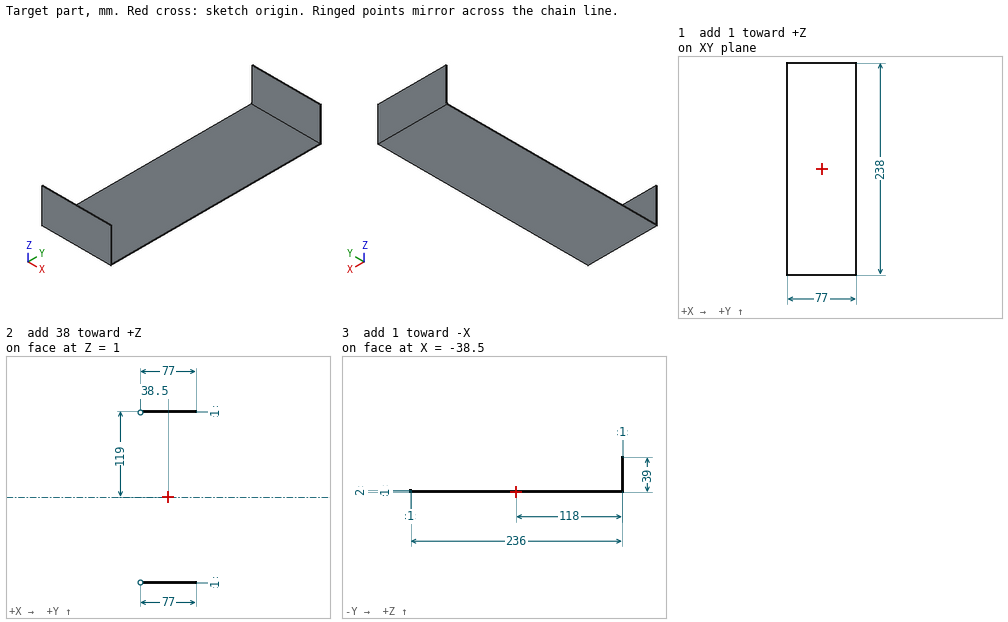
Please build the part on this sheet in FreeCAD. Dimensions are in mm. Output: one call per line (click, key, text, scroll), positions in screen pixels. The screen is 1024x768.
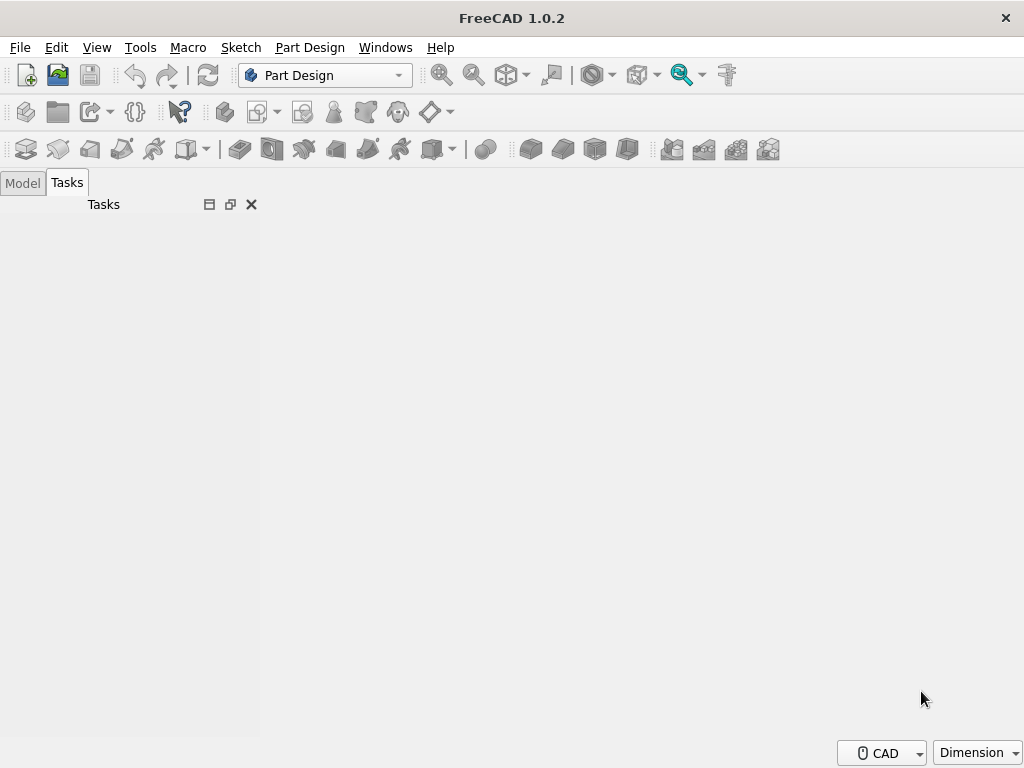
click(26, 76)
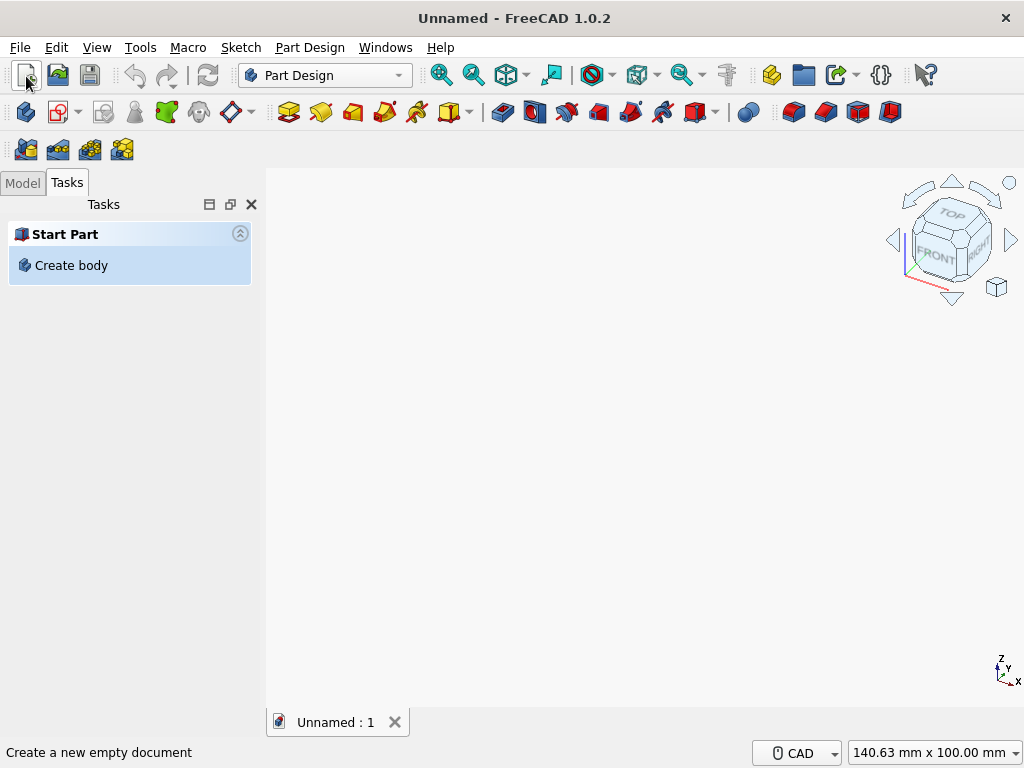
click(58, 112)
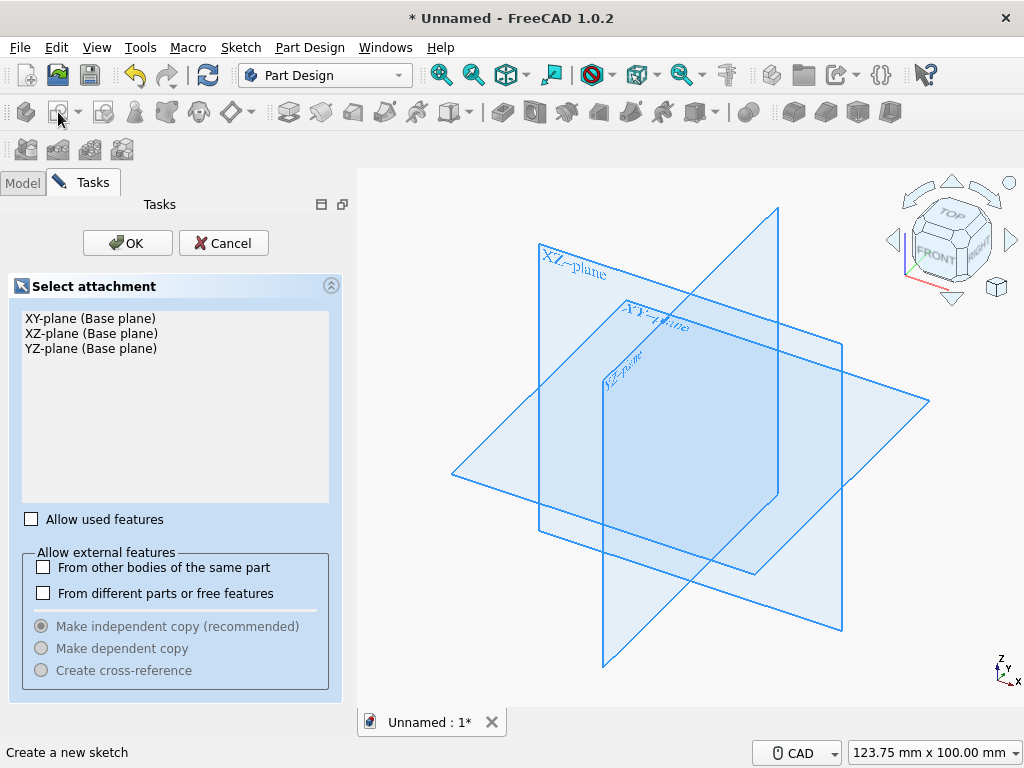
click(82, 318)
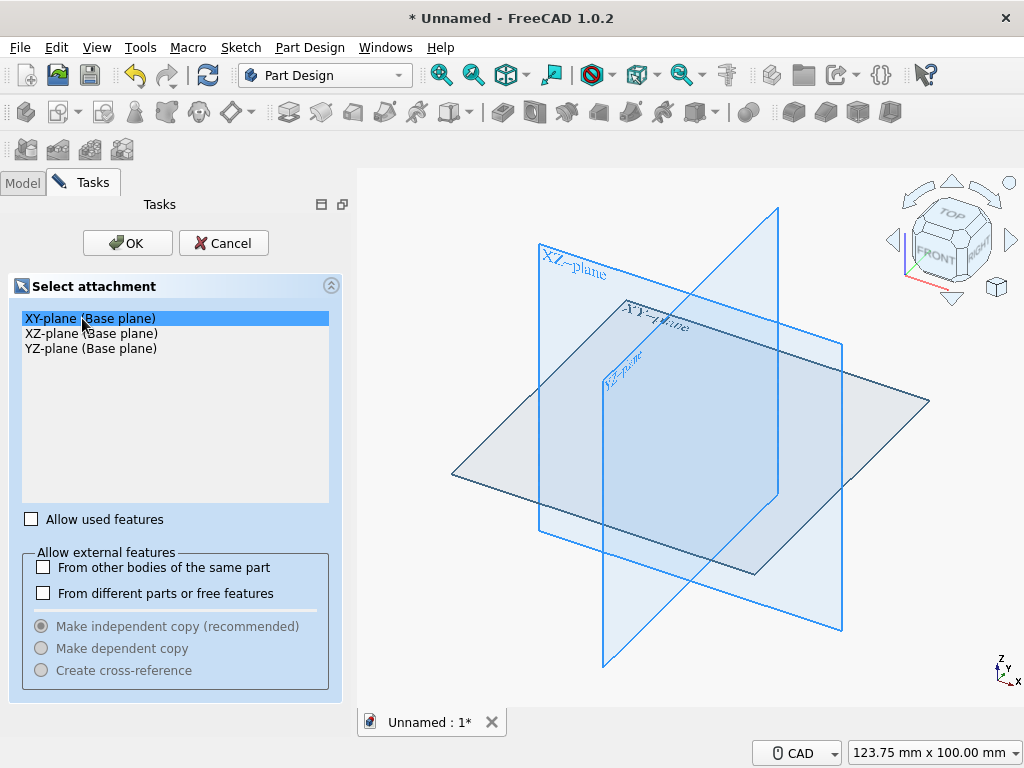
click(128, 243)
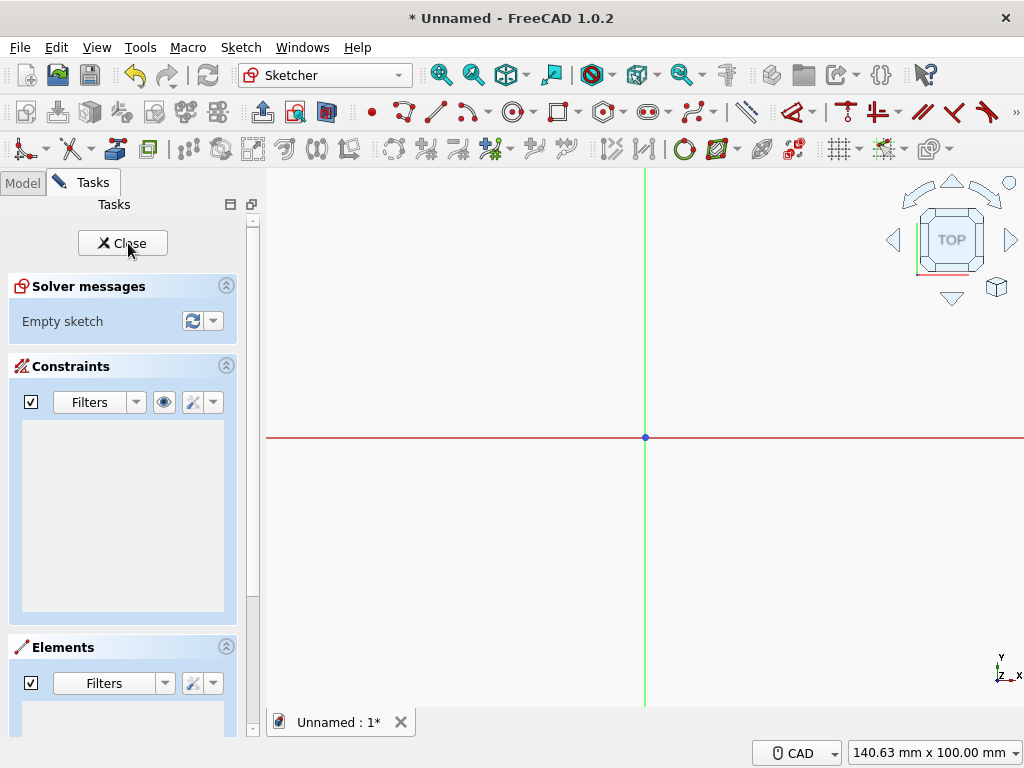
scroll(554, 438, down, 7)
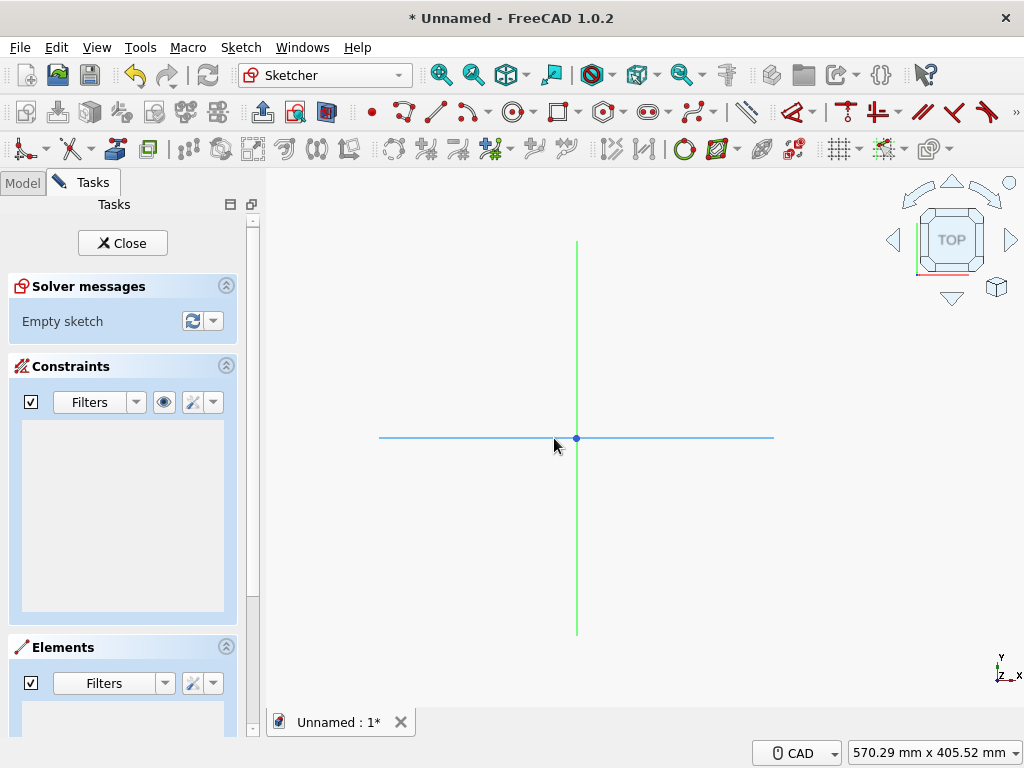
key(g)
key(v)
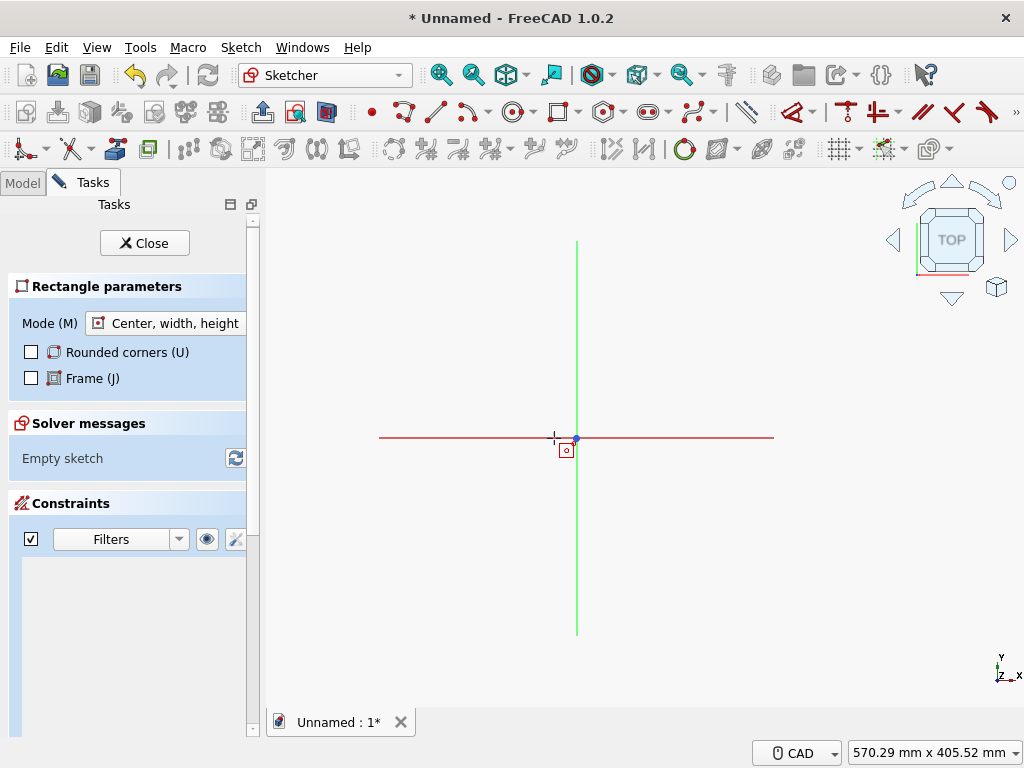
click(577, 438)
move(628, 280)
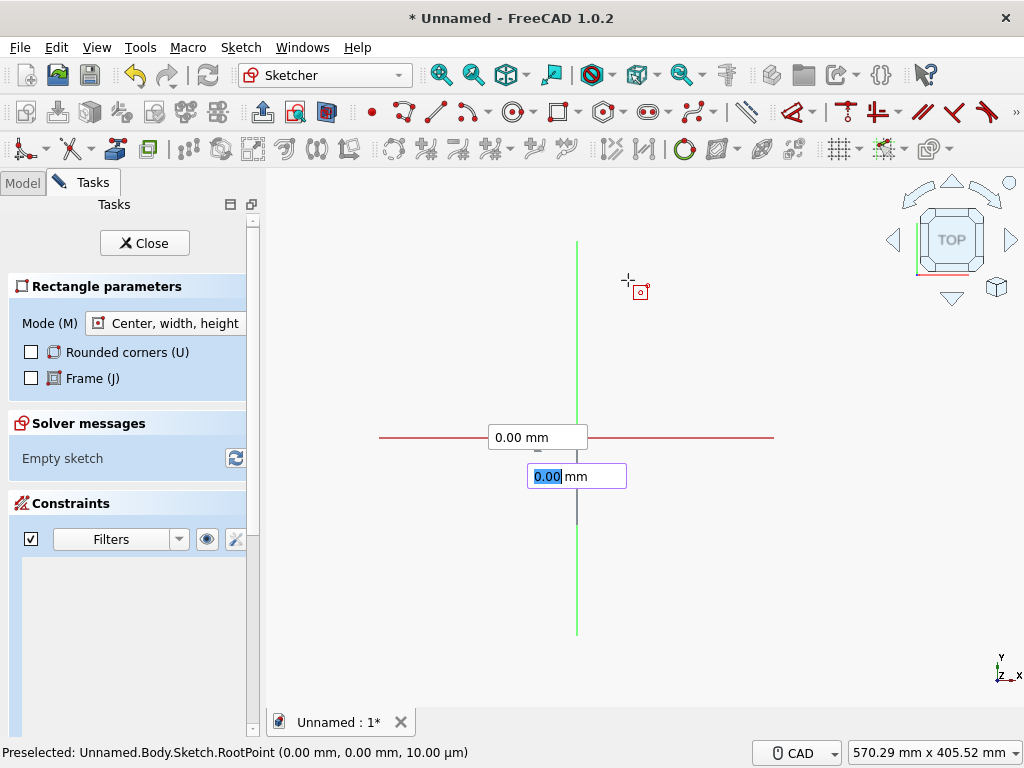
text(77)
key(Tab)
text(238)
key(Return)
key(Escape)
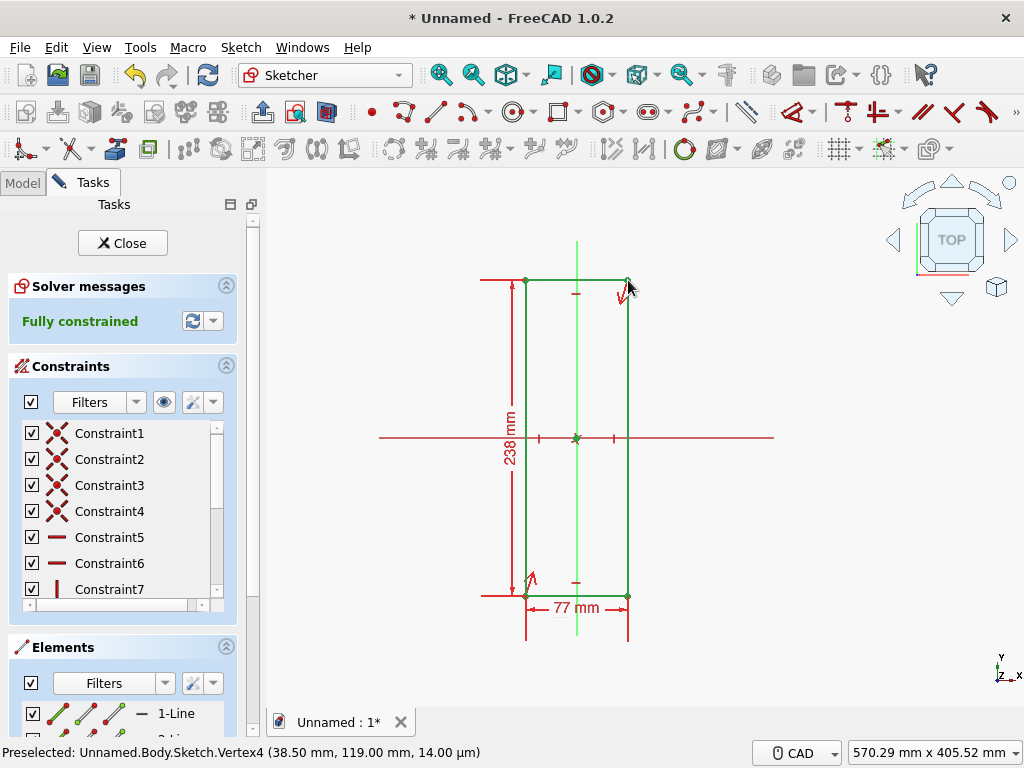
click(123, 243)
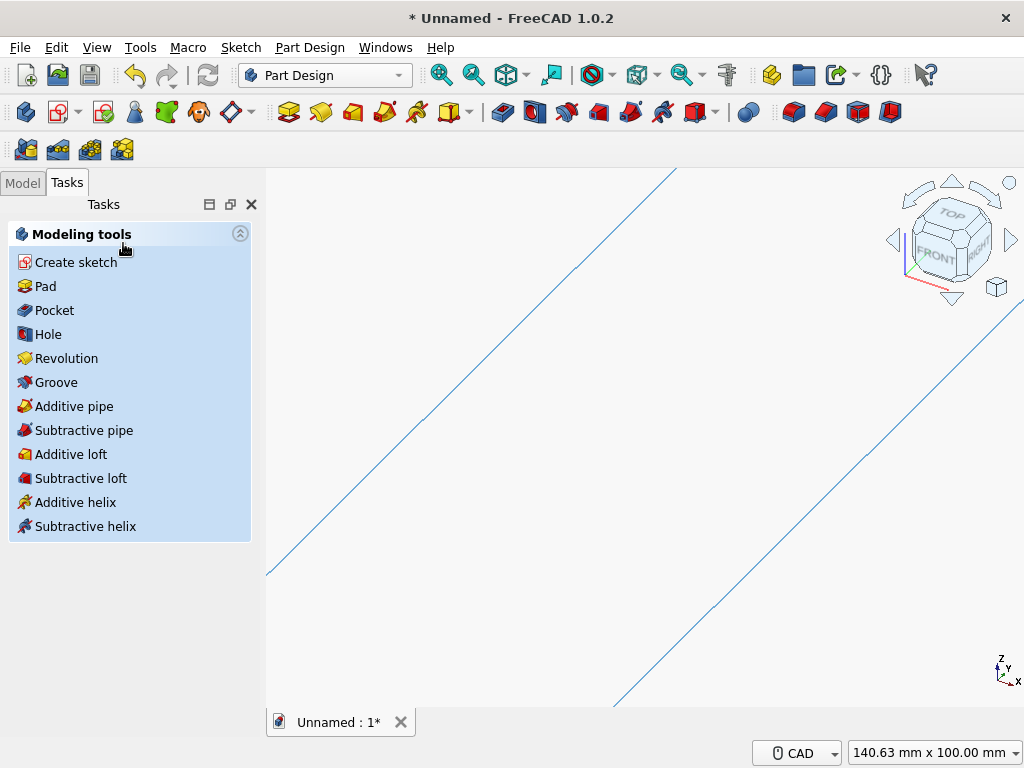
click(290, 112)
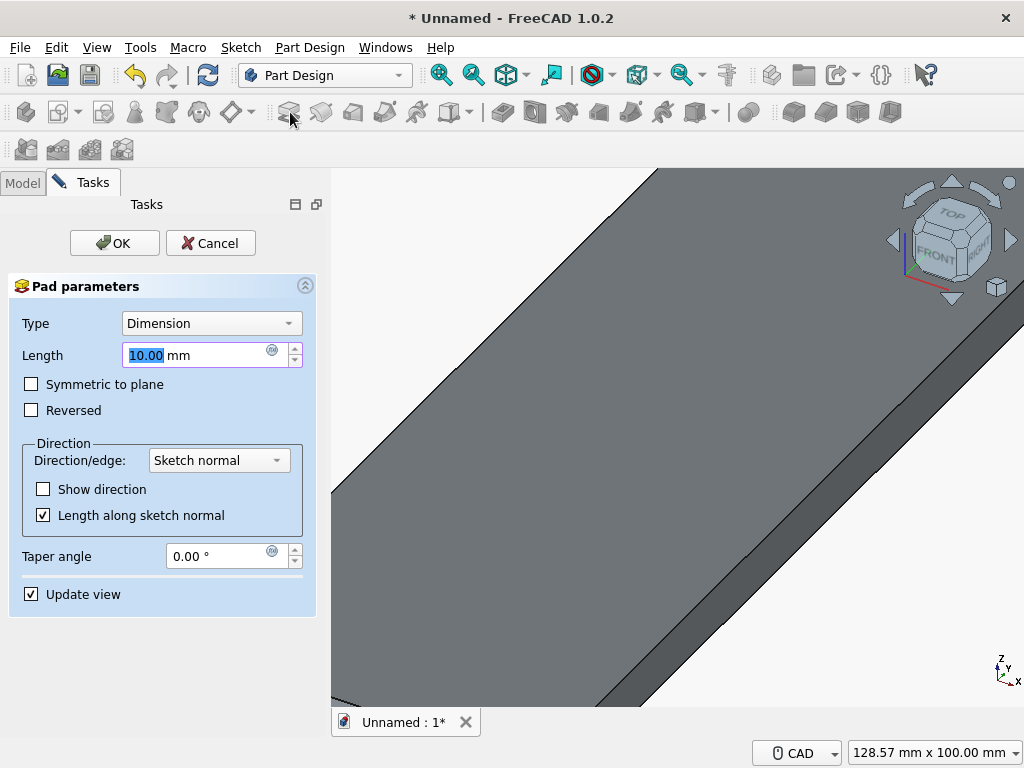
text(1)
key(Tab)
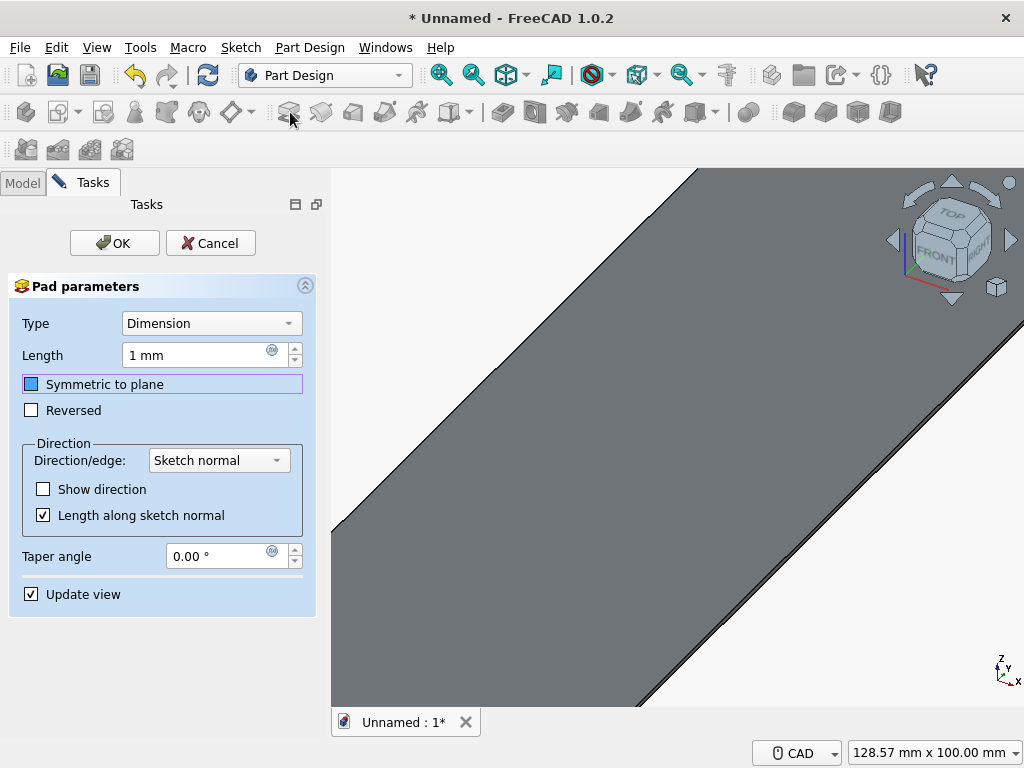
click(115, 243)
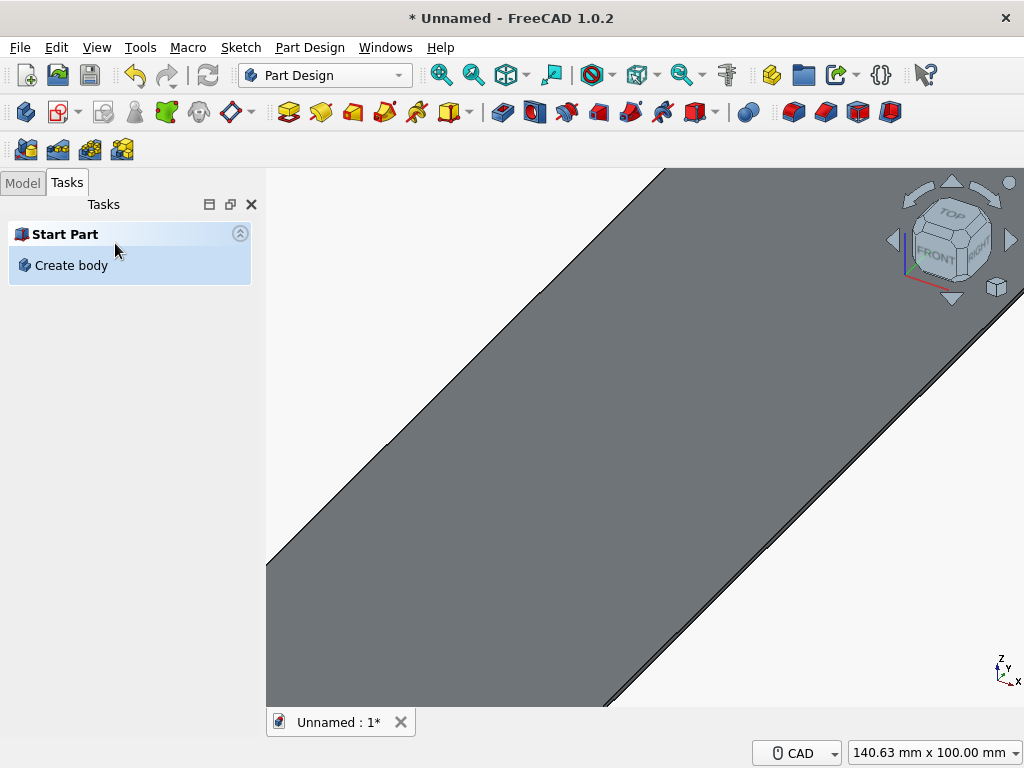
click(442, 76)